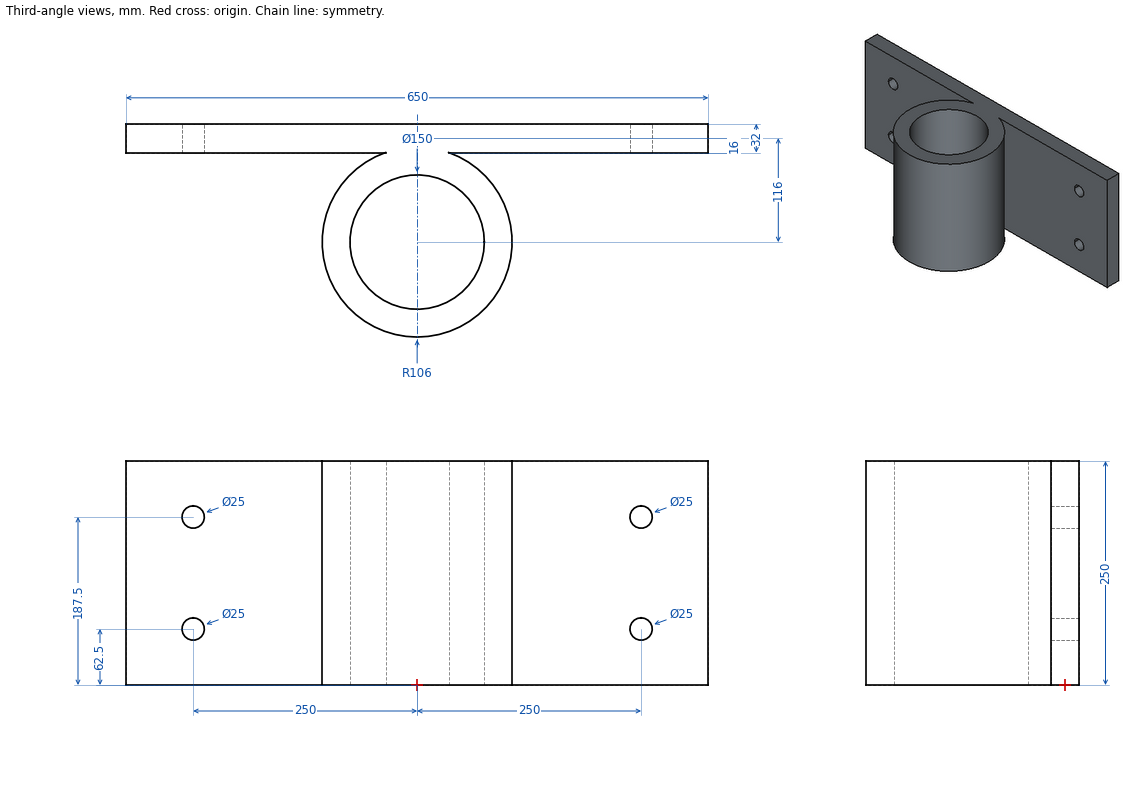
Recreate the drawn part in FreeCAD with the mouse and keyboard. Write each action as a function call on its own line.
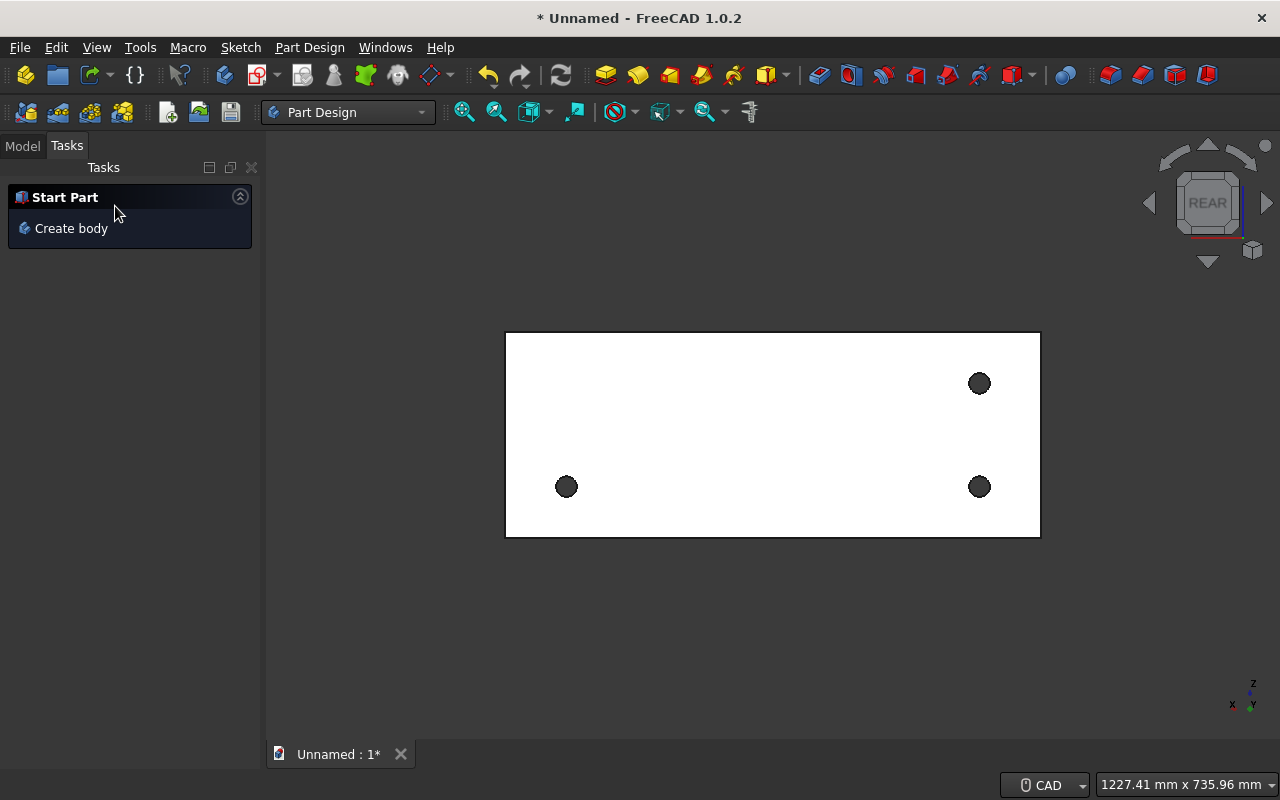
click(696, 434)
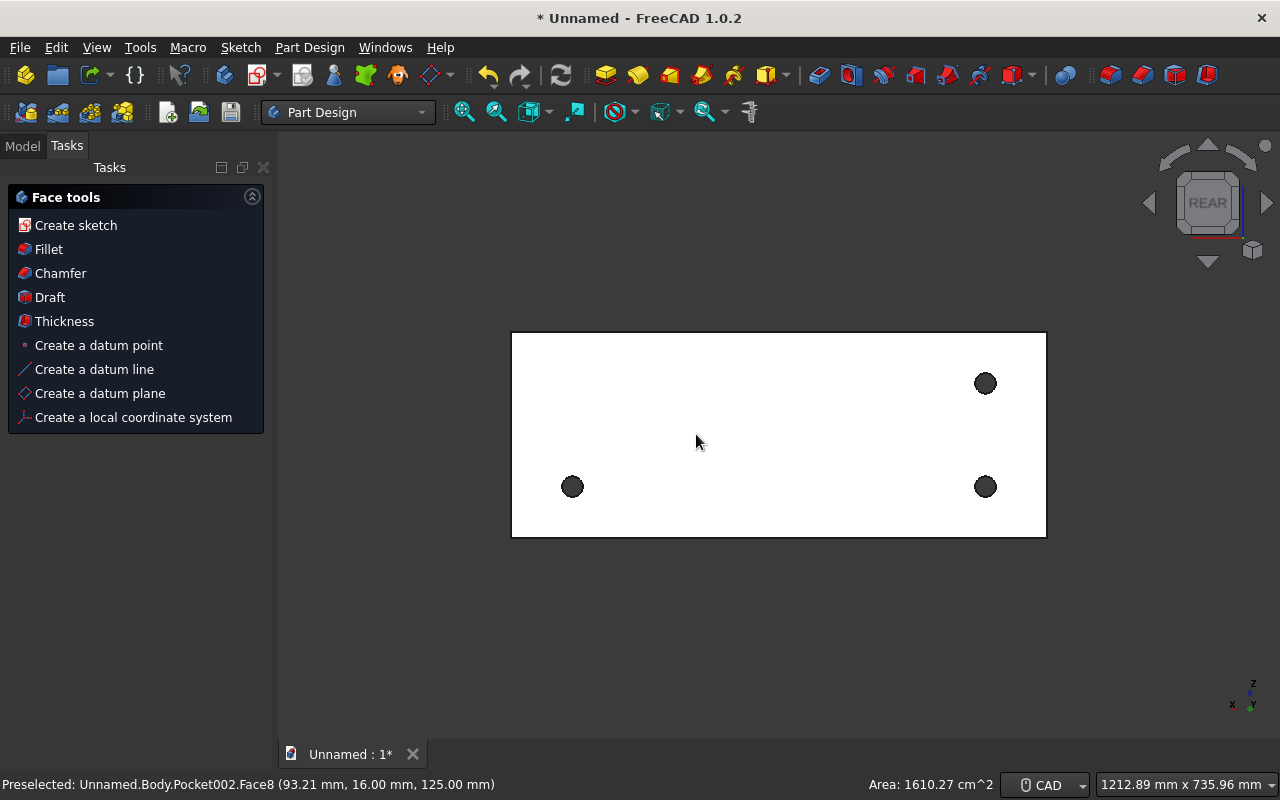
click(258, 76)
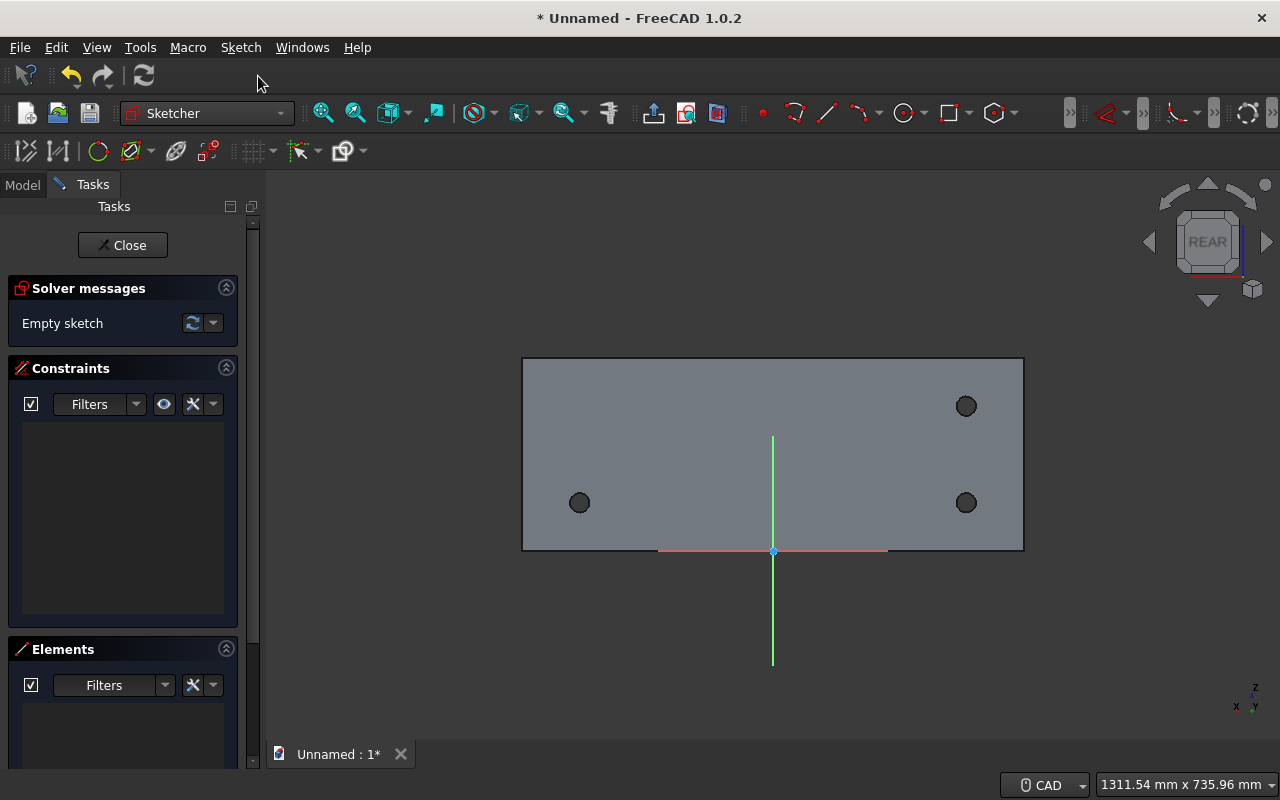
scroll(573, 404, up, 15)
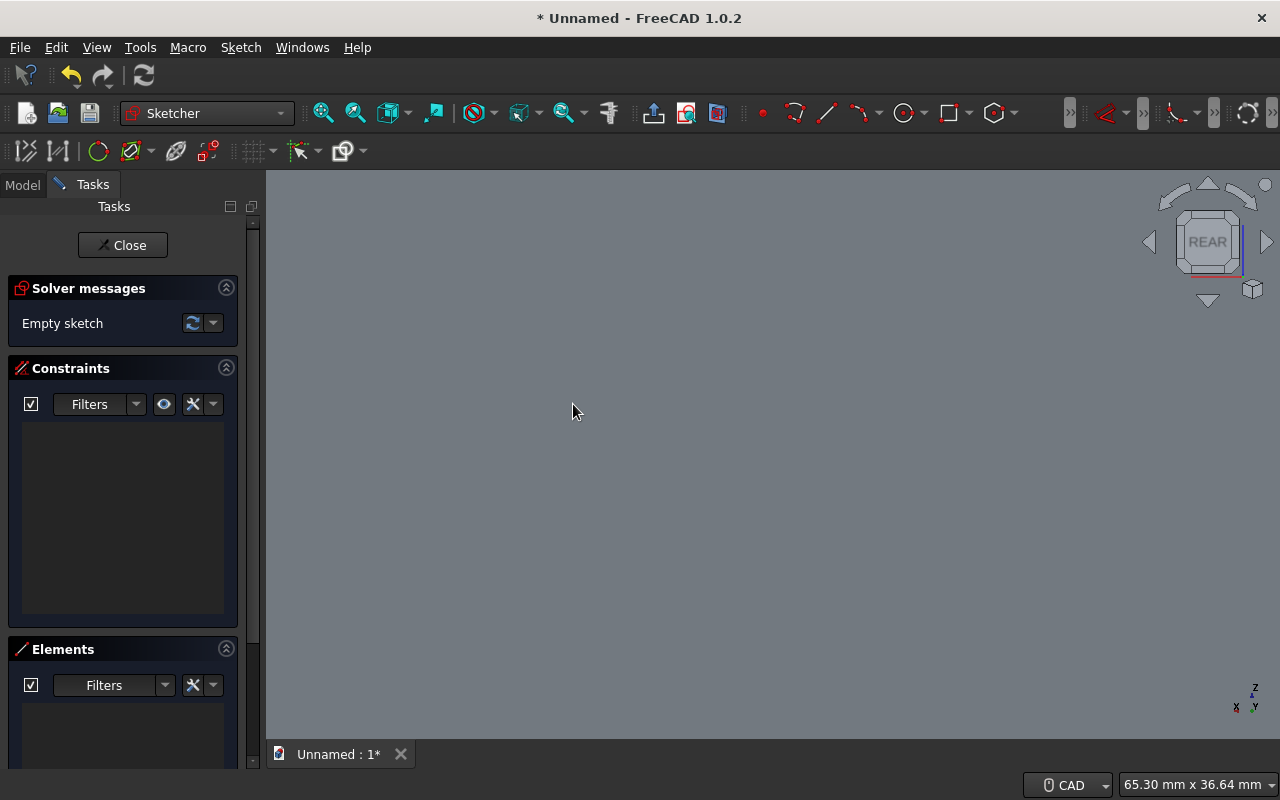
key(g)
key(c)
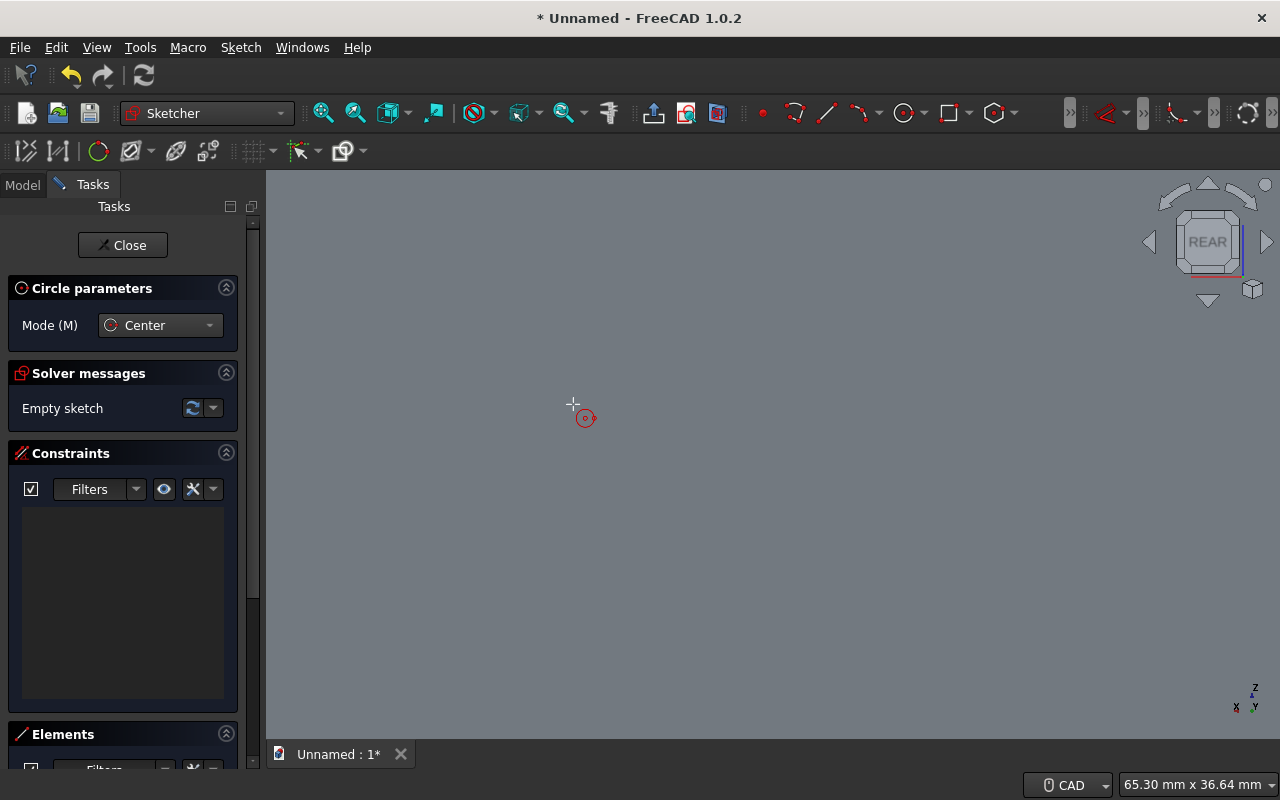
click(702, 440)
click(839, 303)
key(Escape)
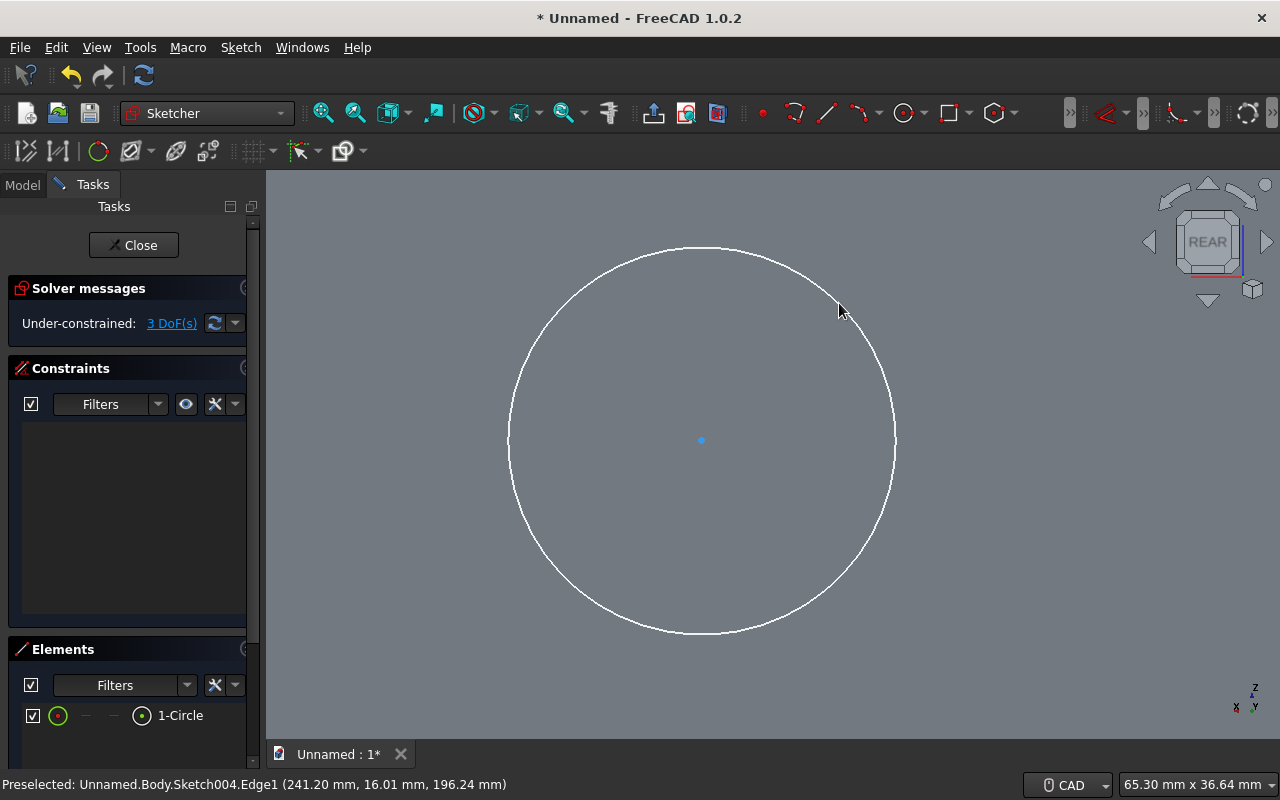
click(1106, 114)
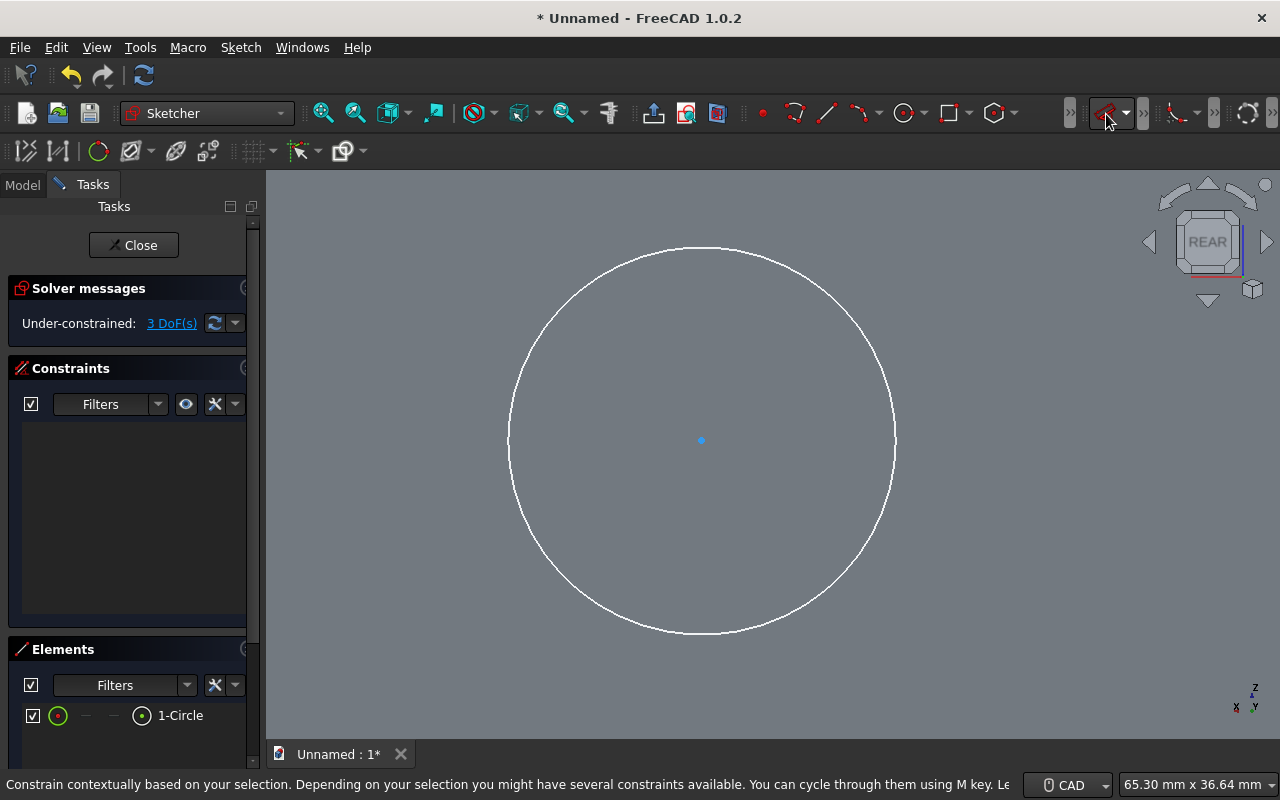
click(839, 304)
click(862, 281)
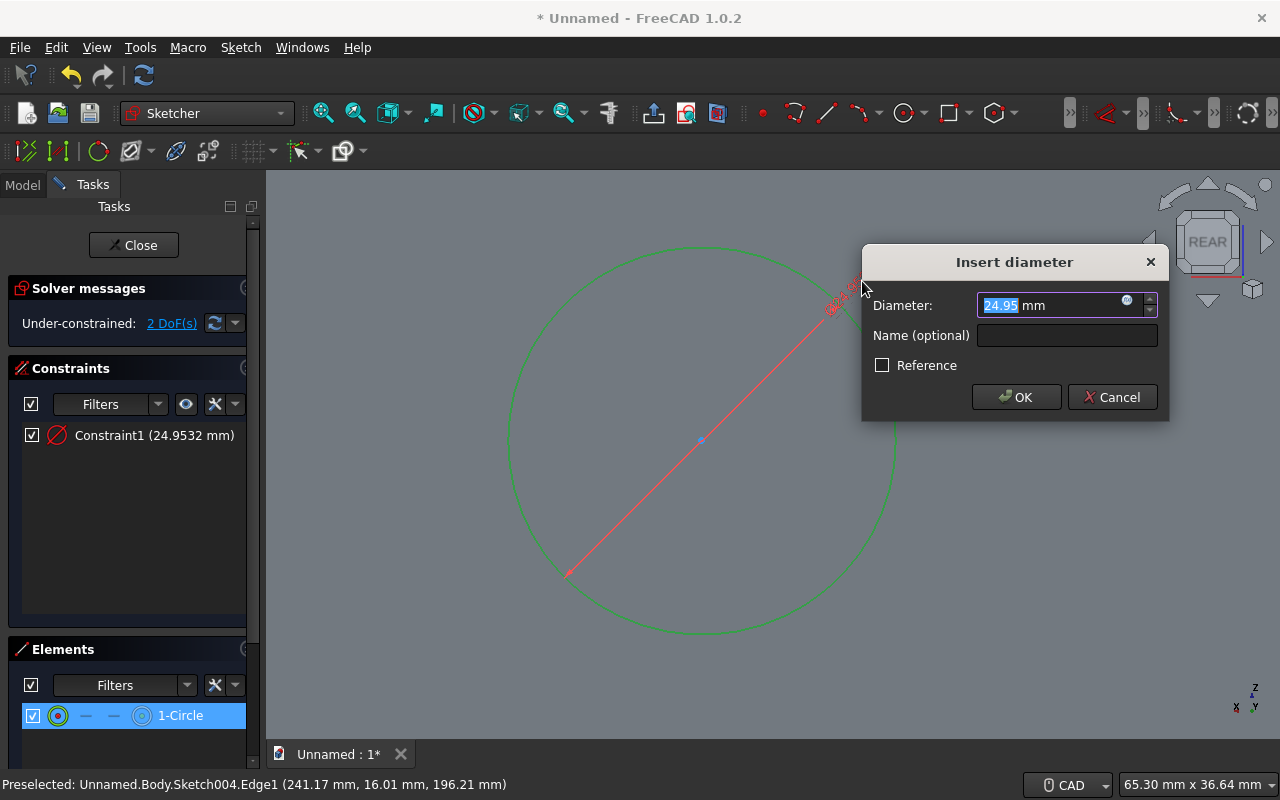
text(25)
key(Return)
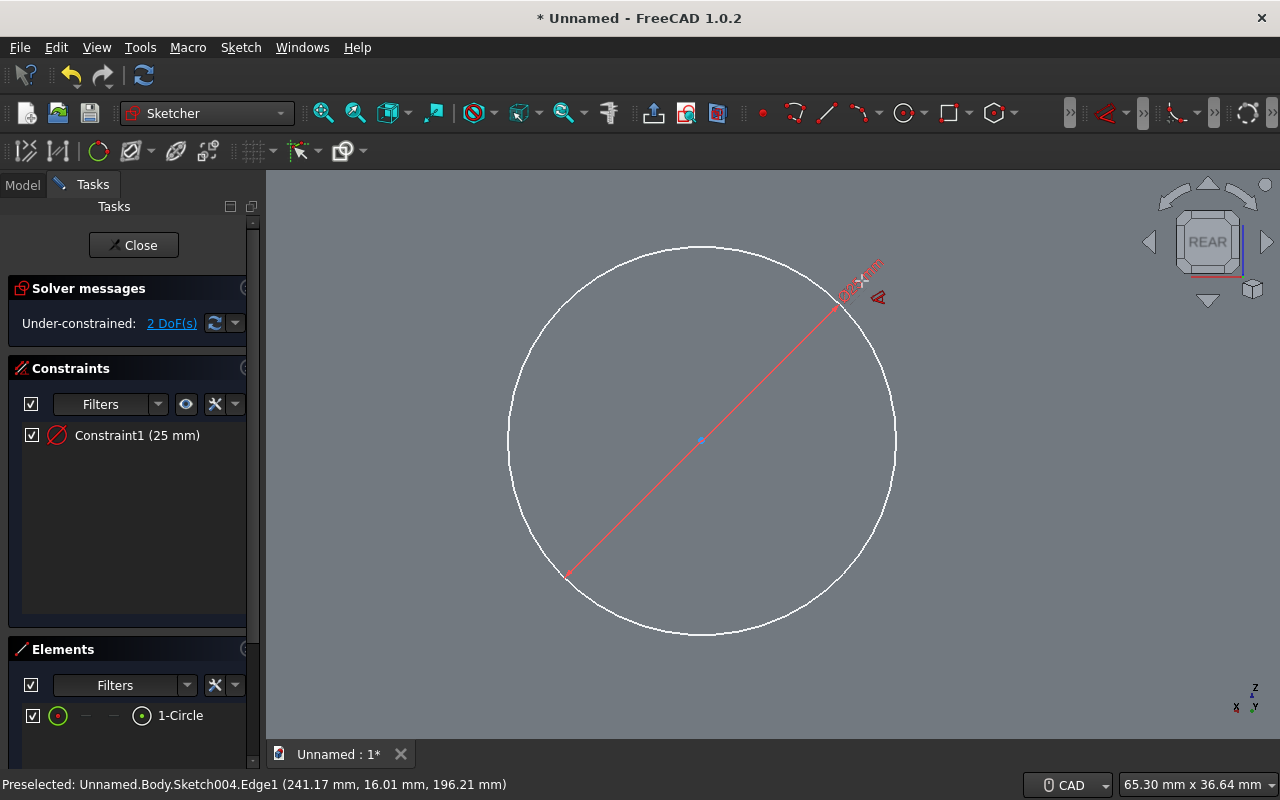
click(702, 441)
click(908, 407)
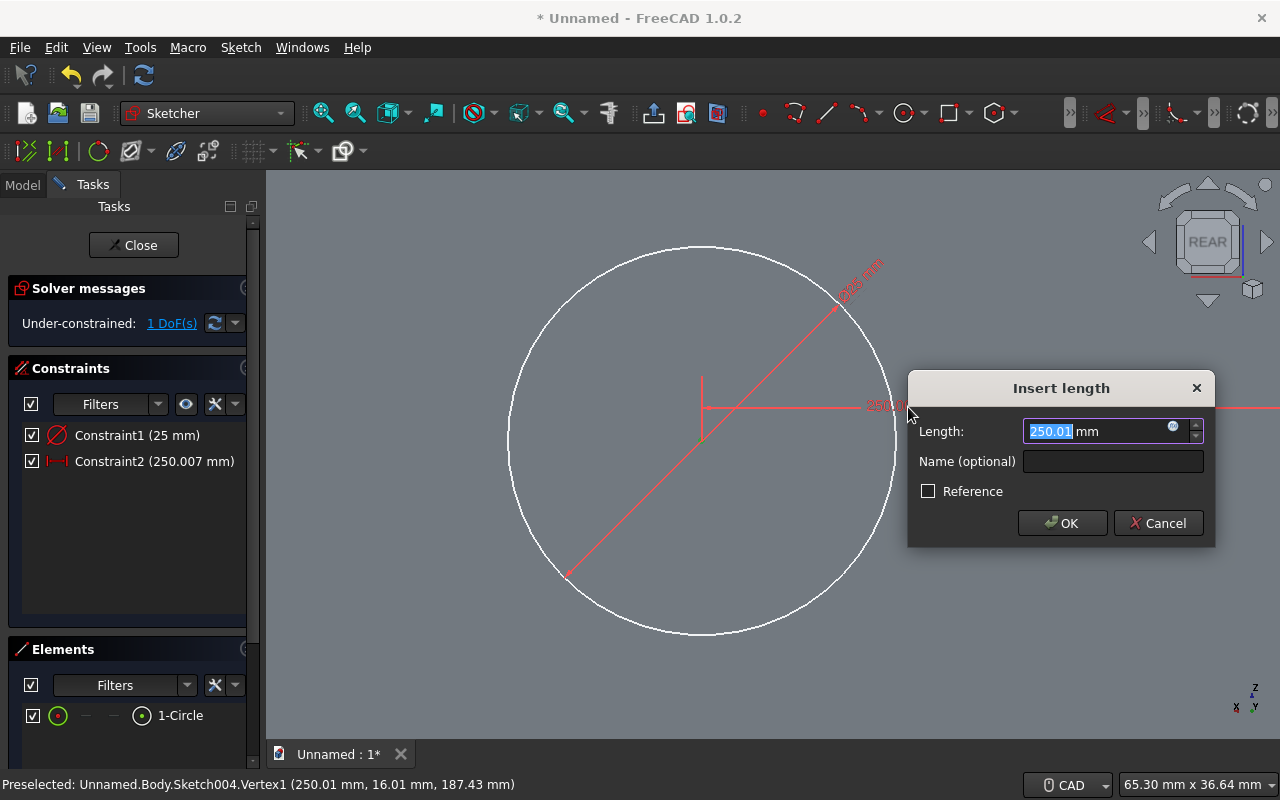
text(250)
key(Return)